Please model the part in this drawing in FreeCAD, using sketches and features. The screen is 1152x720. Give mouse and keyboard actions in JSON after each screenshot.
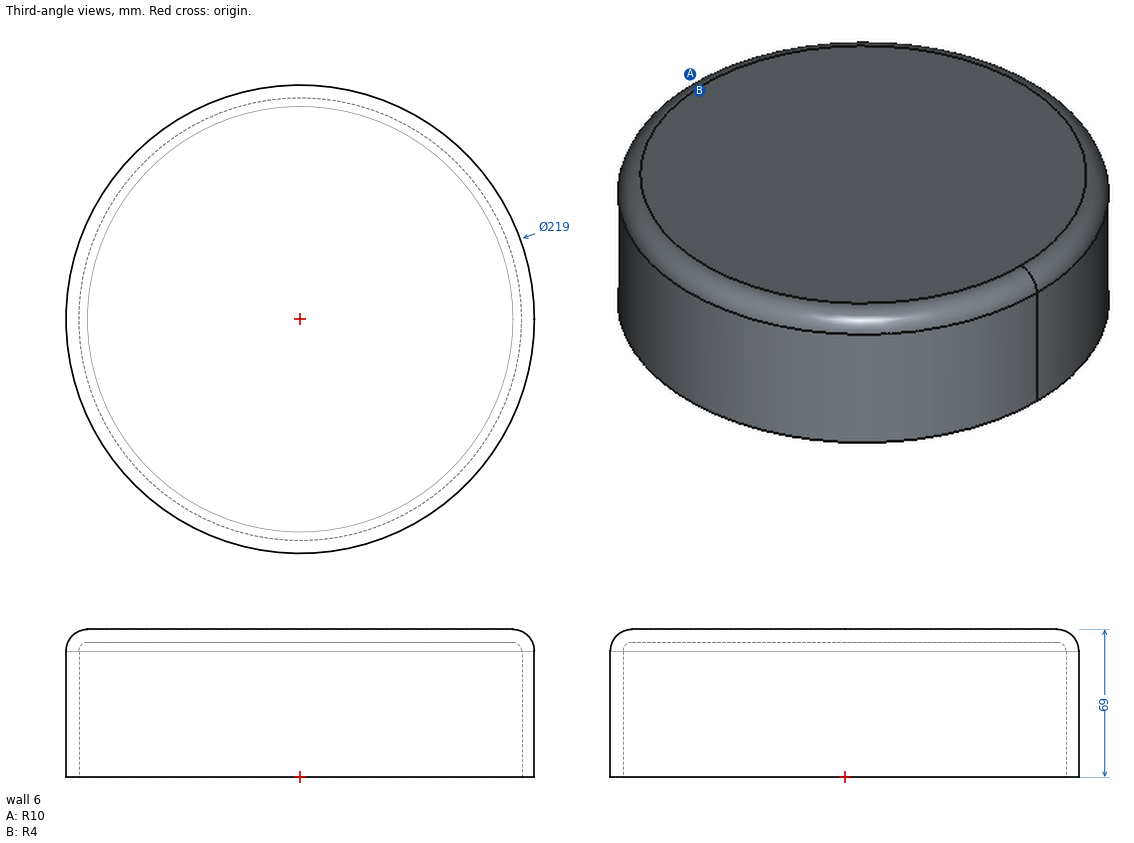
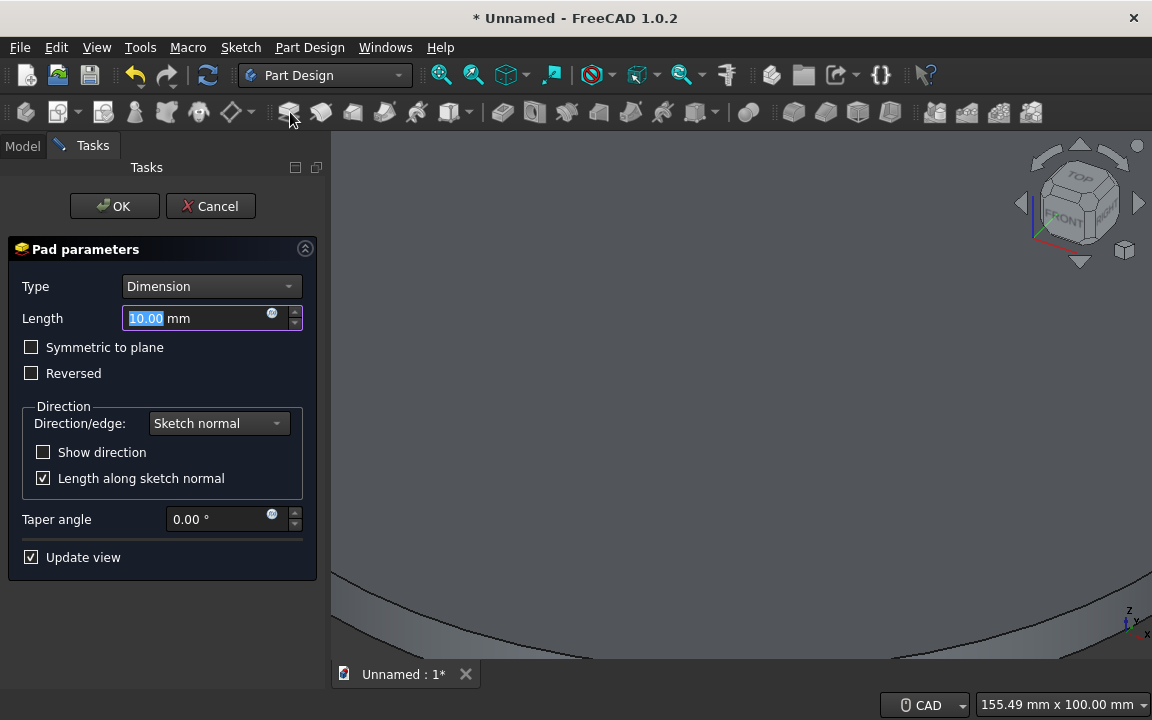
{"action": "type", "text": "69"}
{"action": "key", "text": "Tab"}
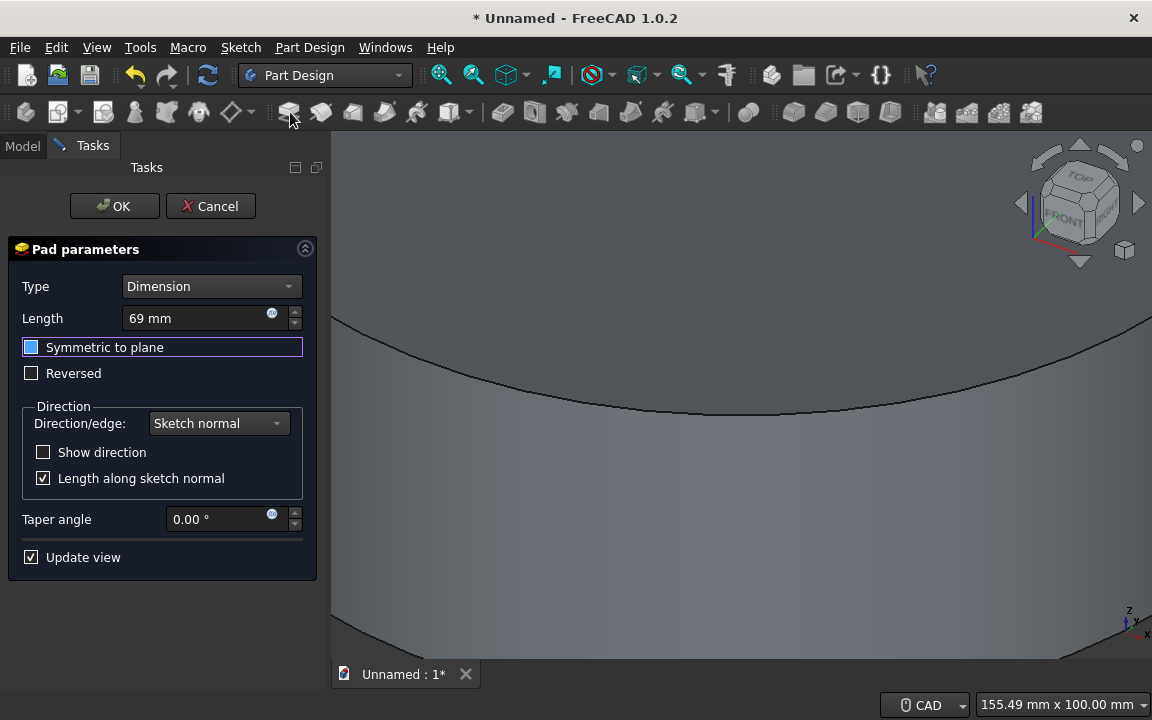
{"action": "left_click", "coordinate": [115, 206]}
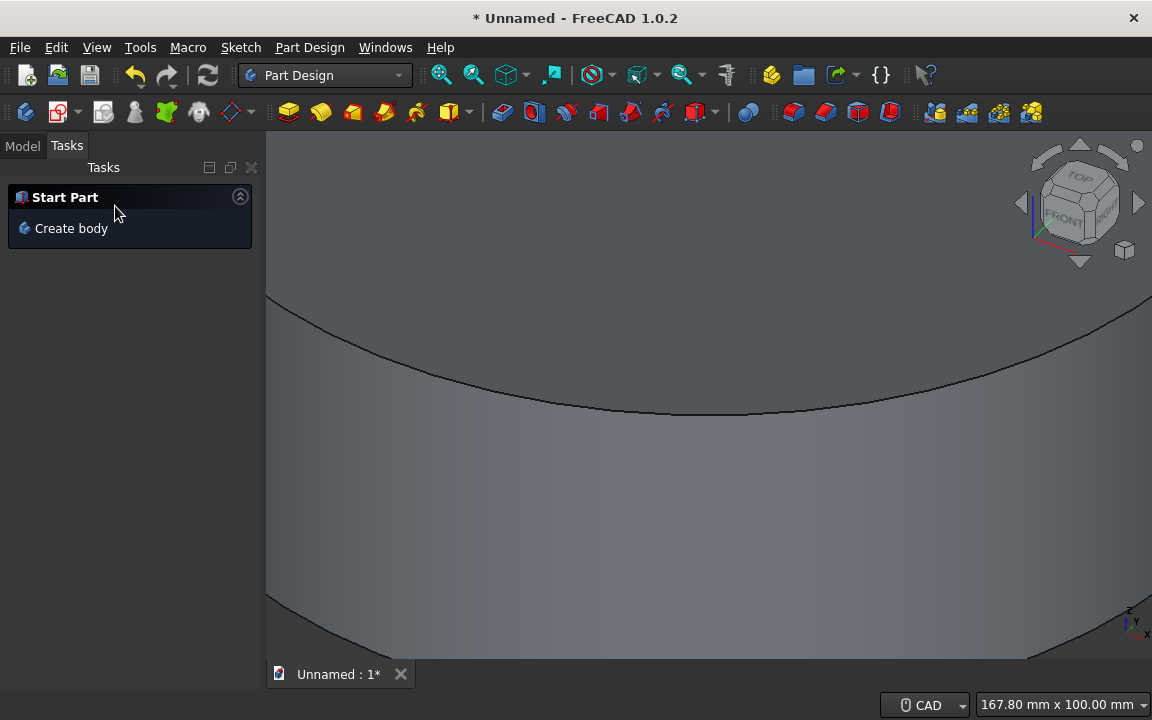
{"action": "left_click", "coordinate": [442, 76]}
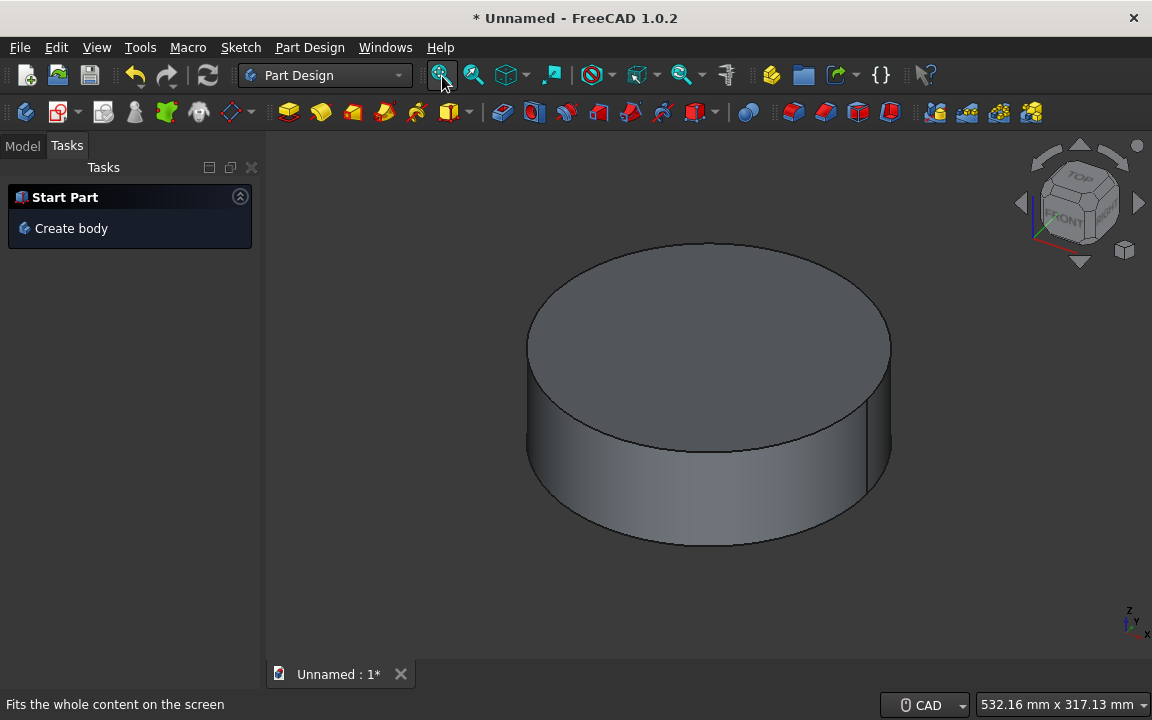
{"action": "key", "text": "0"}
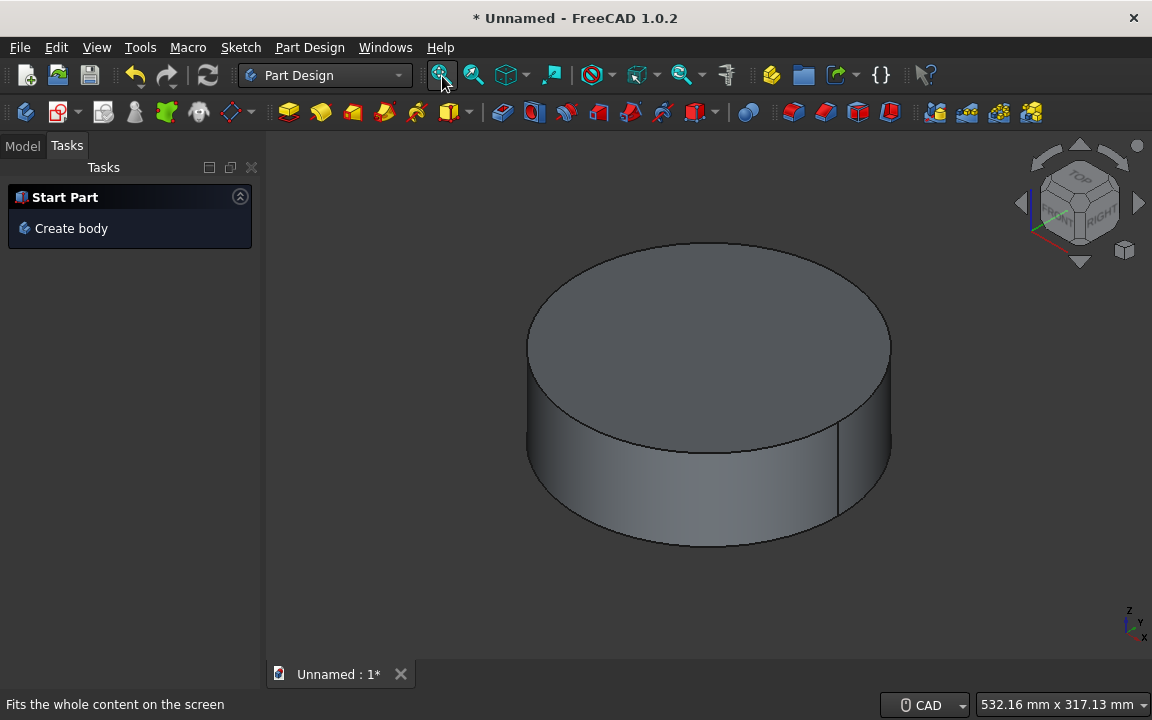
{"action": "key", "text": "2"}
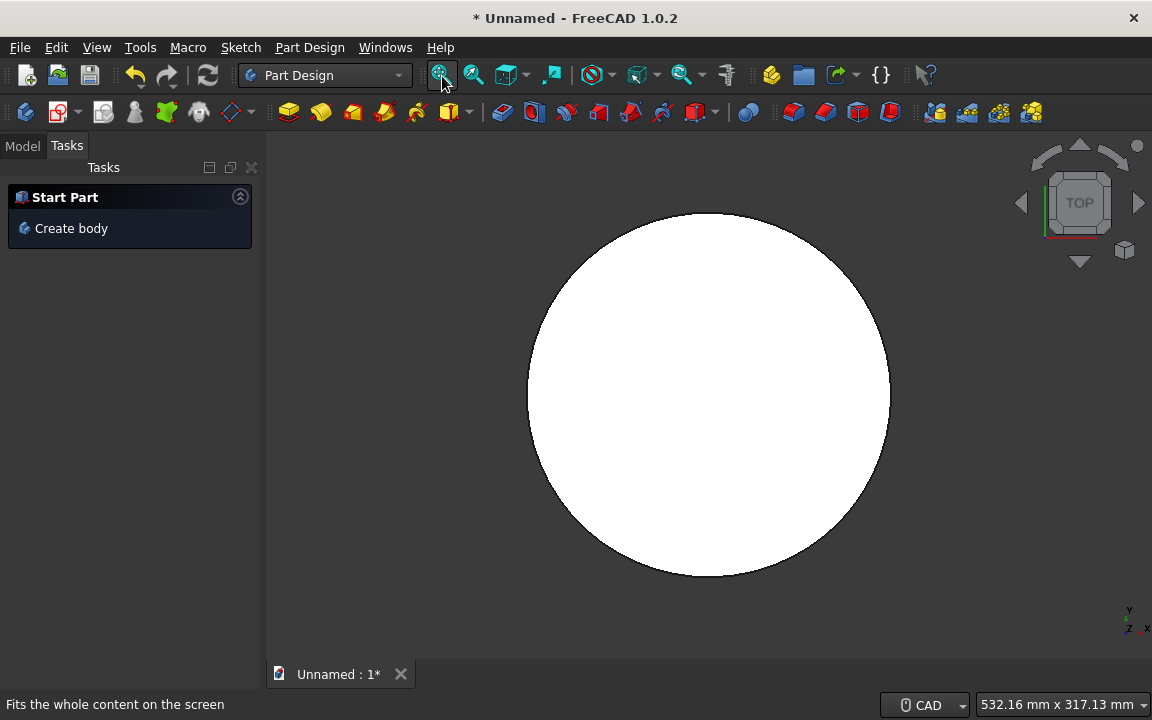
{"action": "key", "text": "1"}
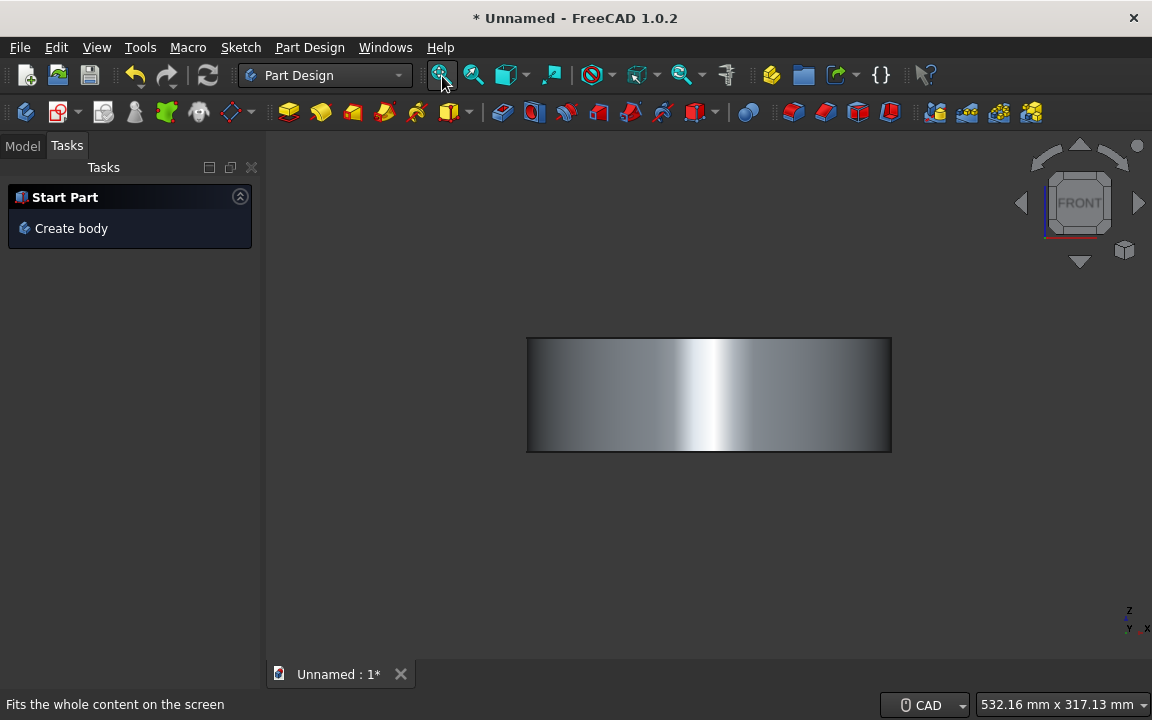
{"action": "key", "text": "v f"}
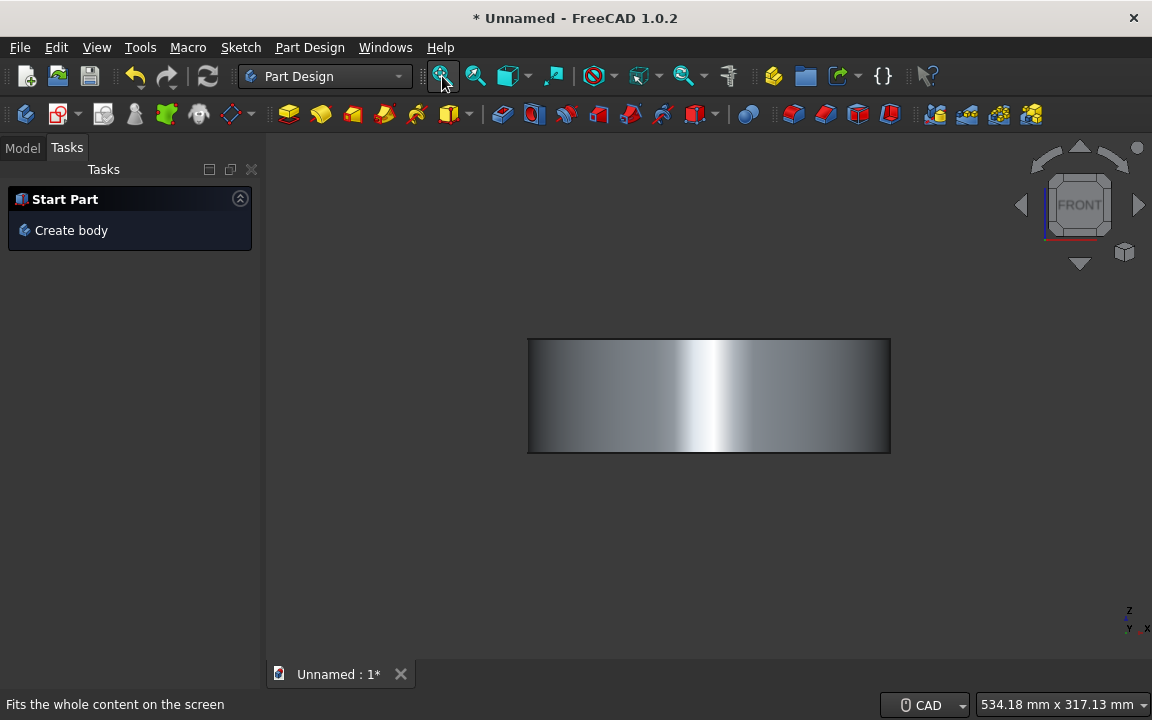
{"action": "key", "text": "3"}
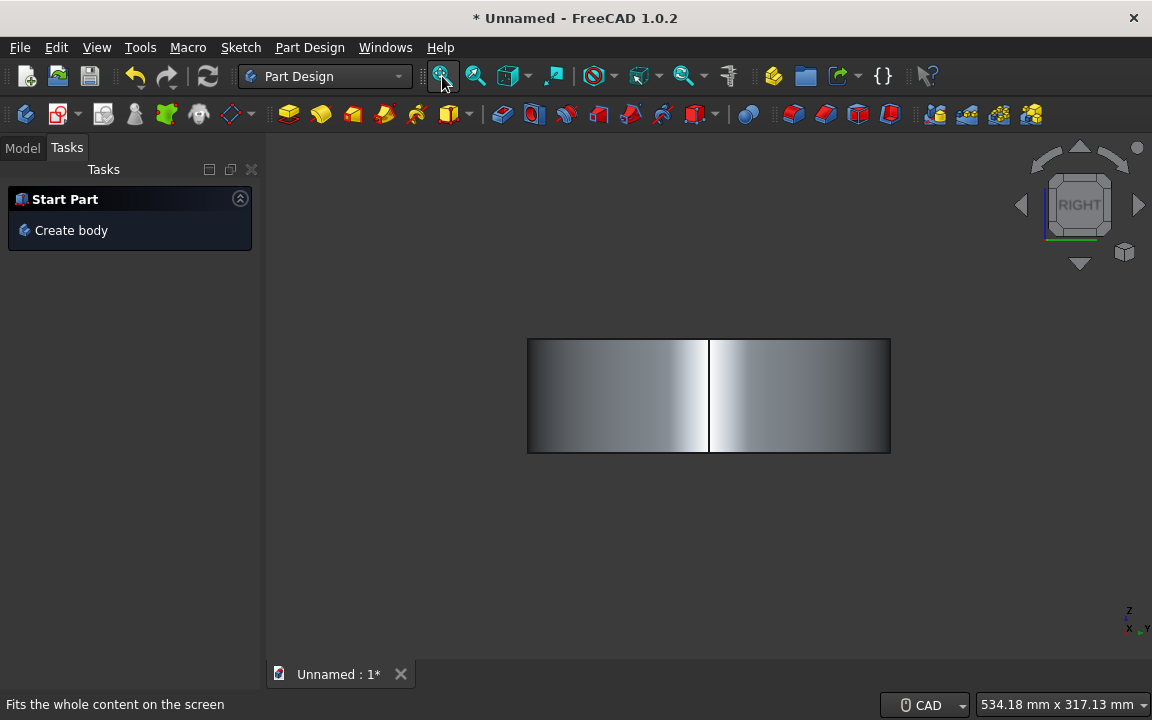
{"action": "key", "text": "v f"}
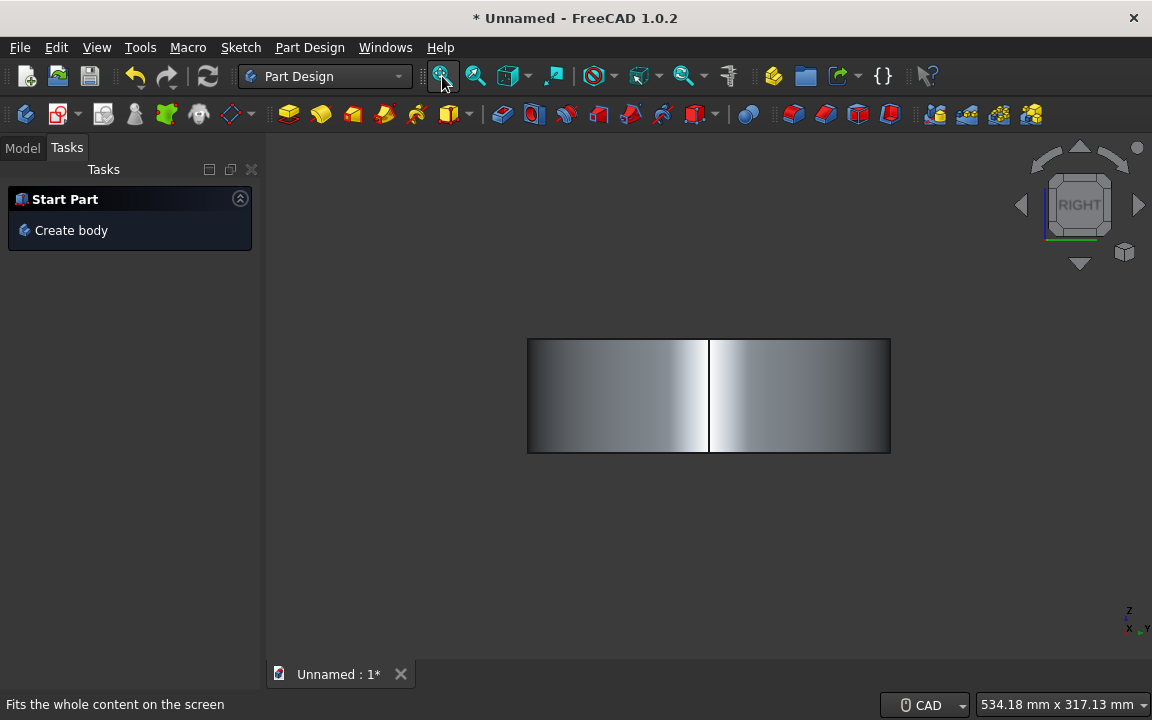
{"action": "key", "text": "5"}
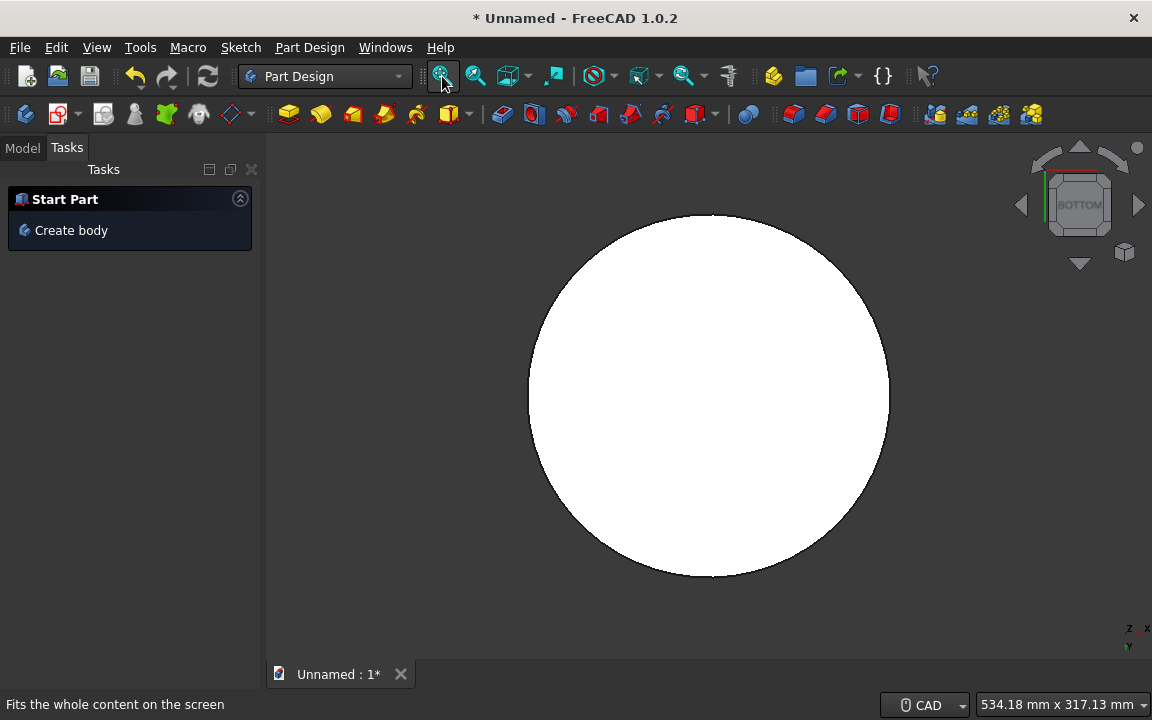
{"action": "left_click", "coordinate": [709, 395]}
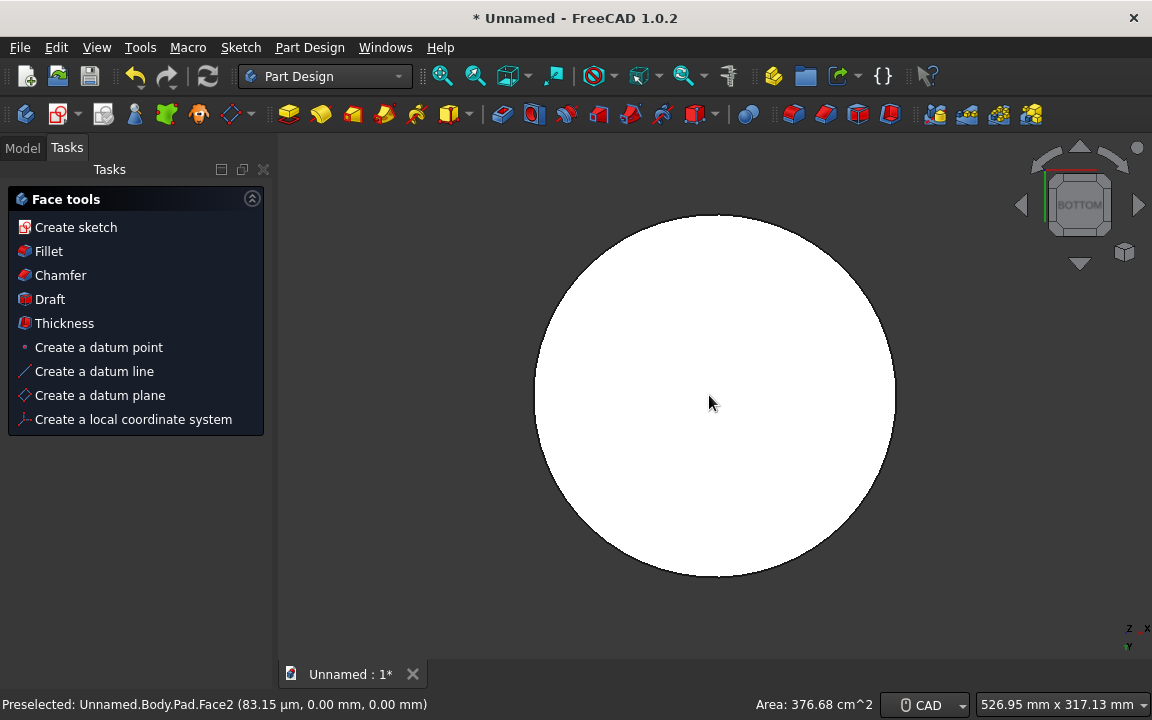
{"action": "left_click", "coordinate": [890, 114]}